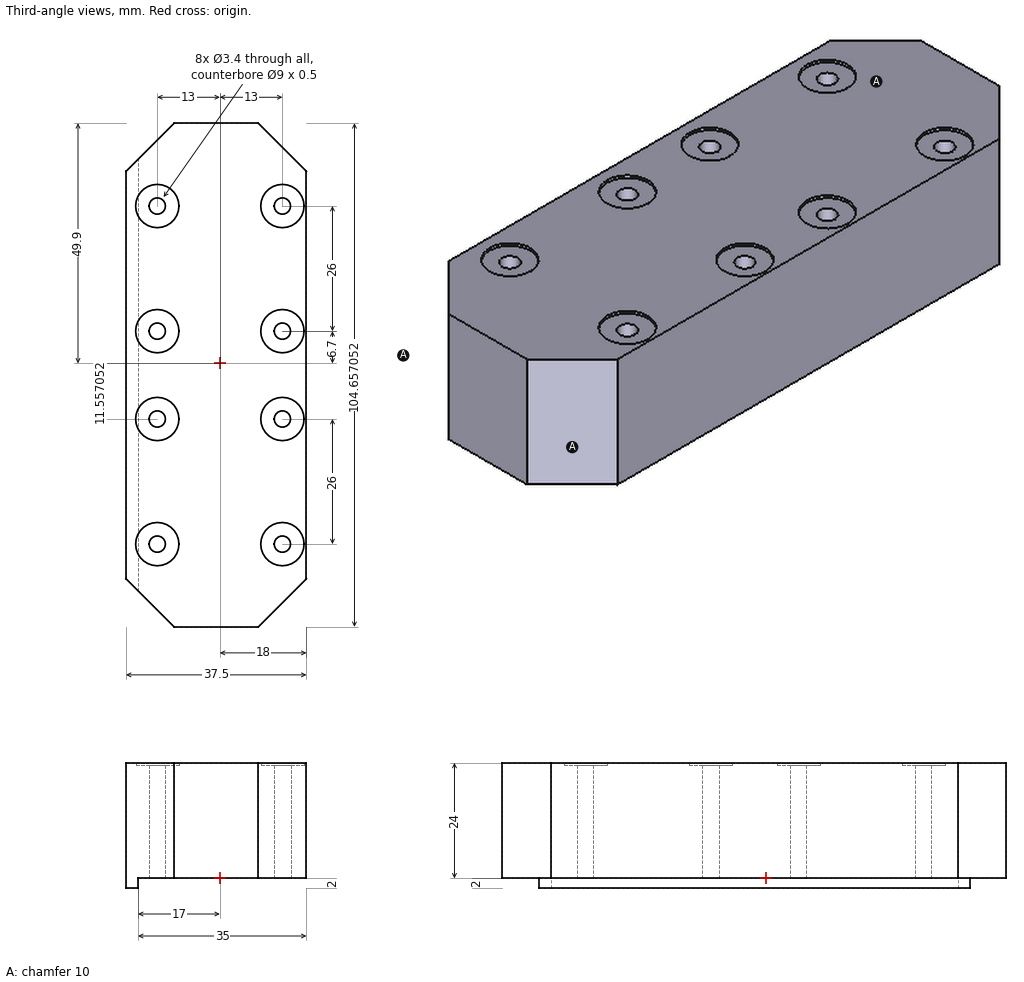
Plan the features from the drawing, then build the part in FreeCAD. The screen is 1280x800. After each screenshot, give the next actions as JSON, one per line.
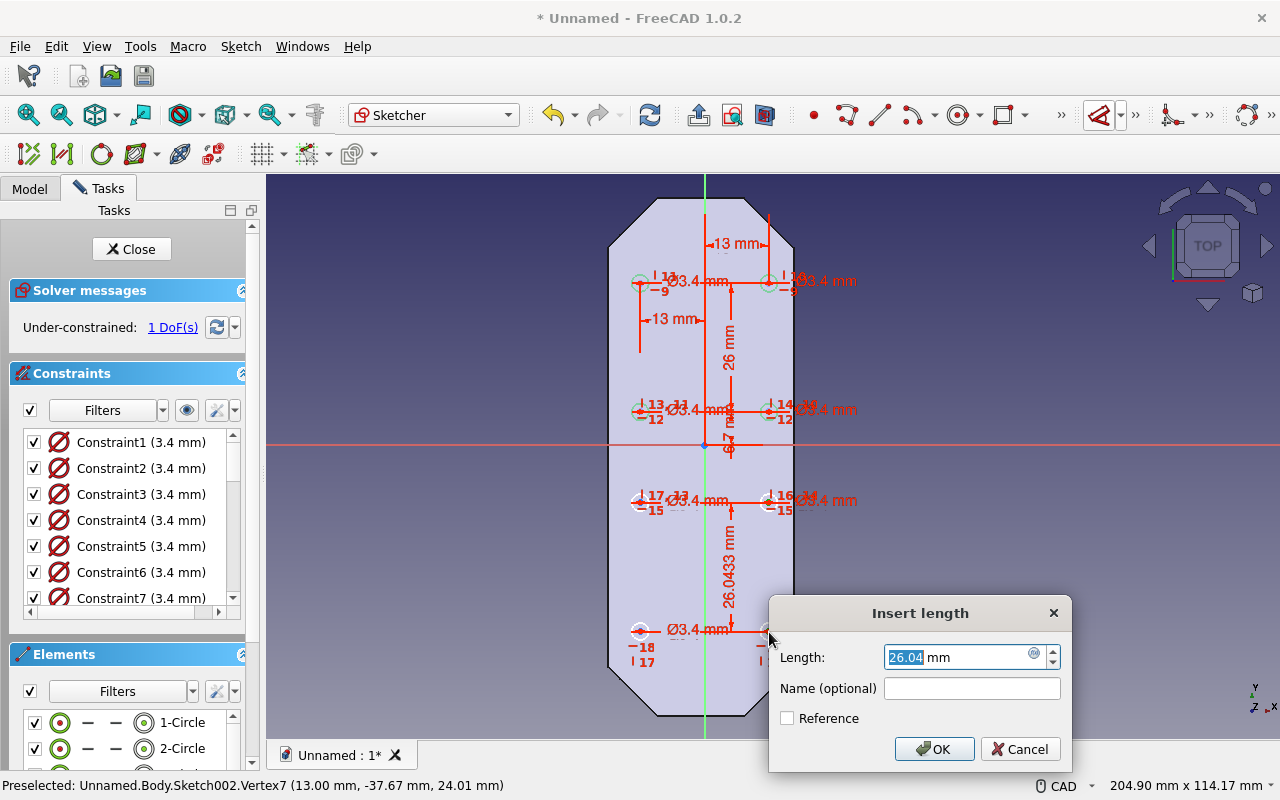
{"action": "type", "text": "26"}
{"action": "key", "text": "Return"}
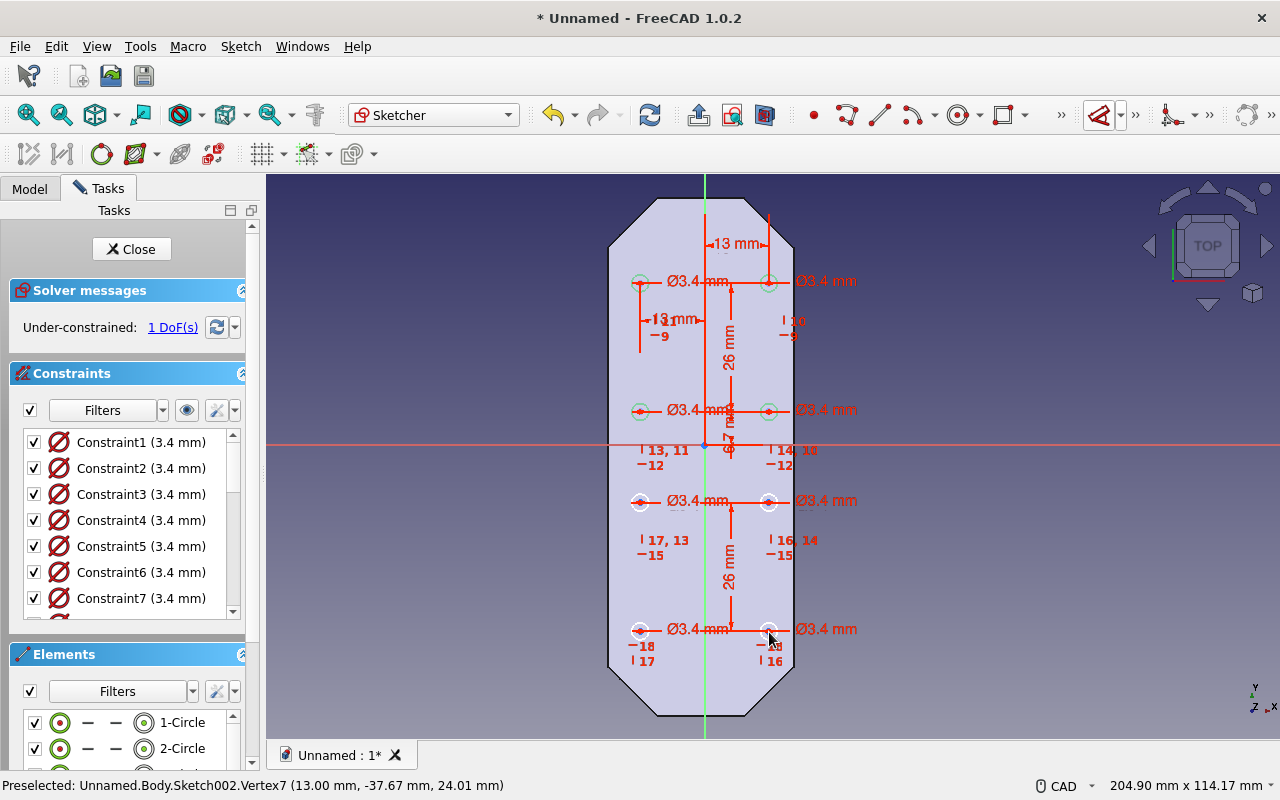
{"action": "left_click", "coordinate": [640, 503]}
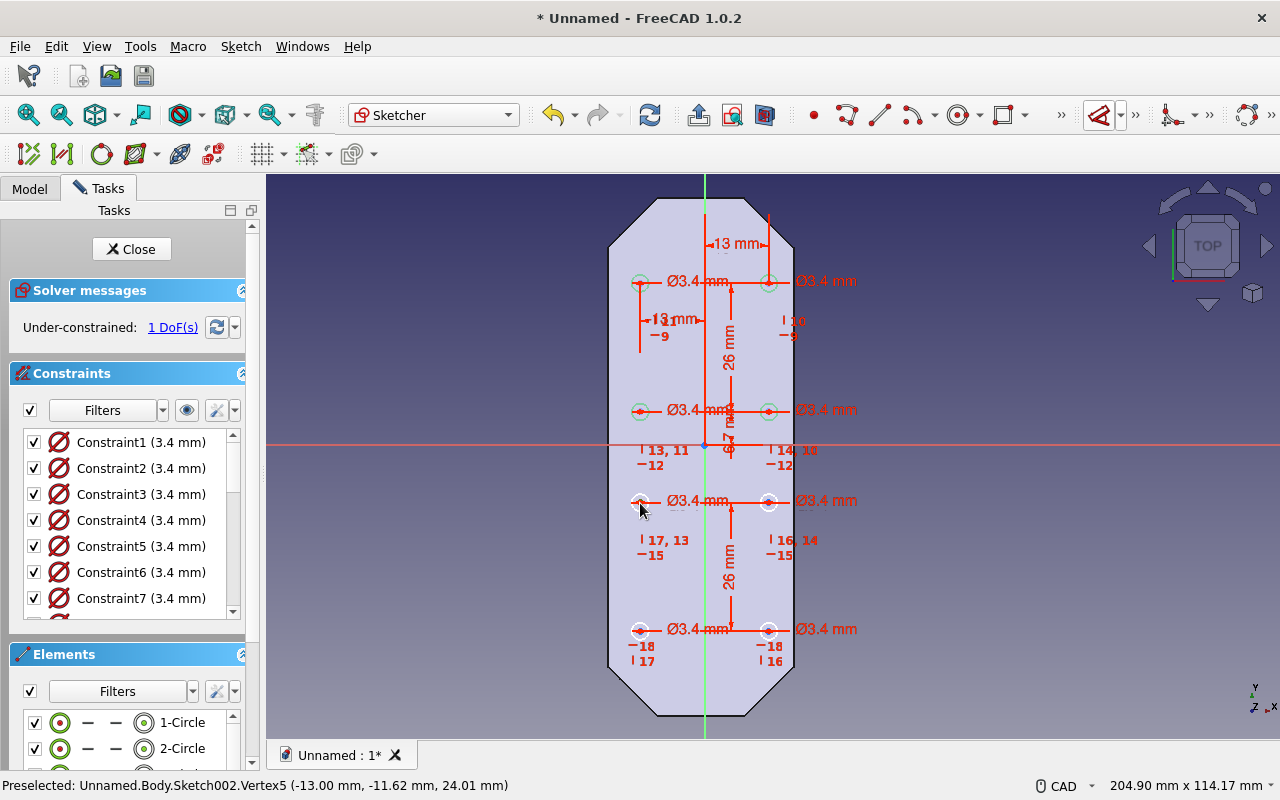
{"action": "left_click", "coordinate": [1120, 116]}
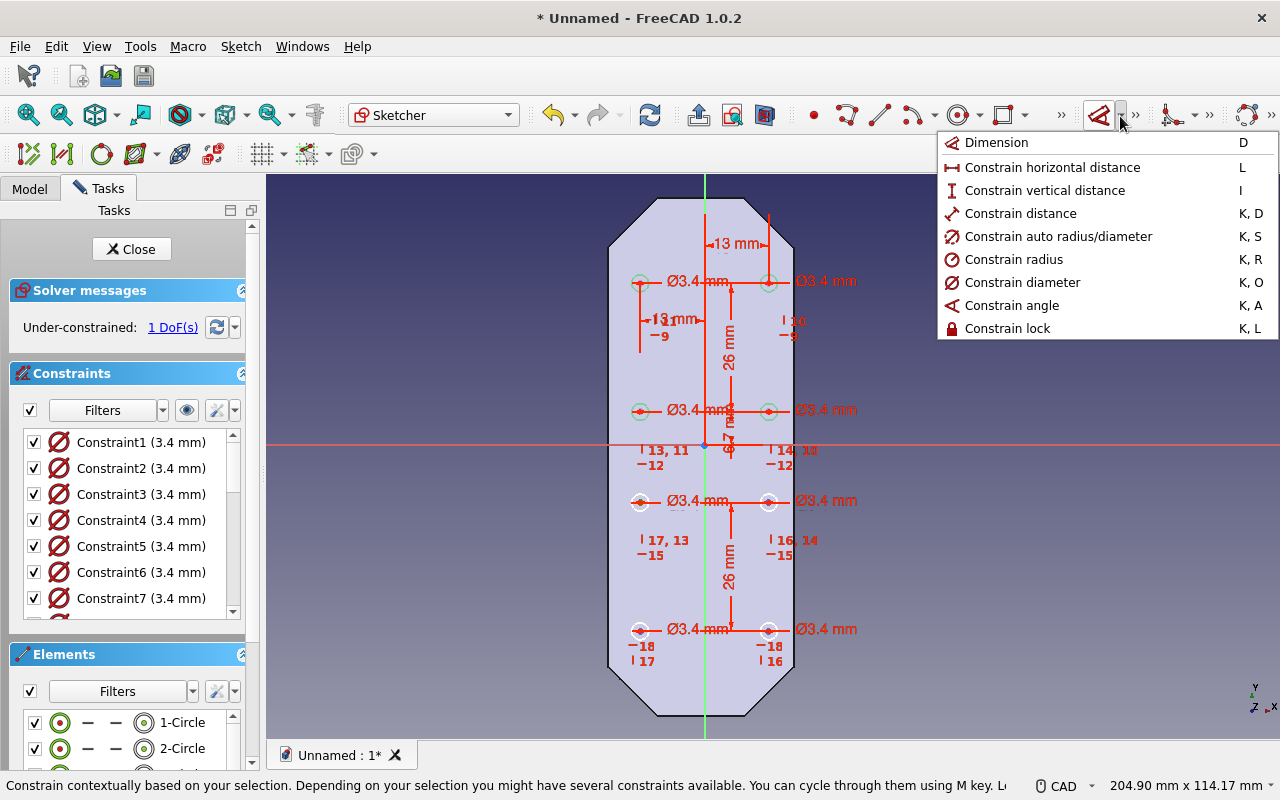
{"action": "left_click", "coordinate": [1108, 190]}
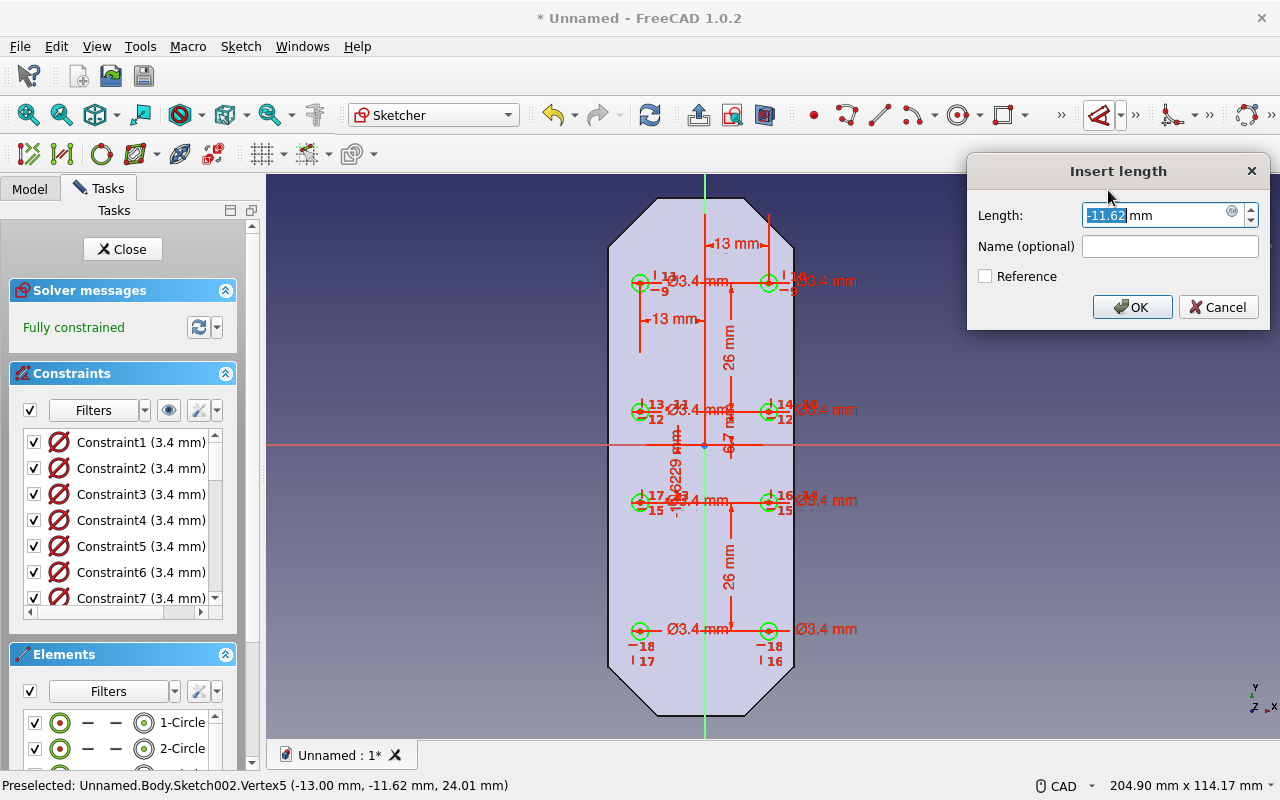
{"action": "type", "text": "-11.557052"}
{"action": "key", "text": "Return"}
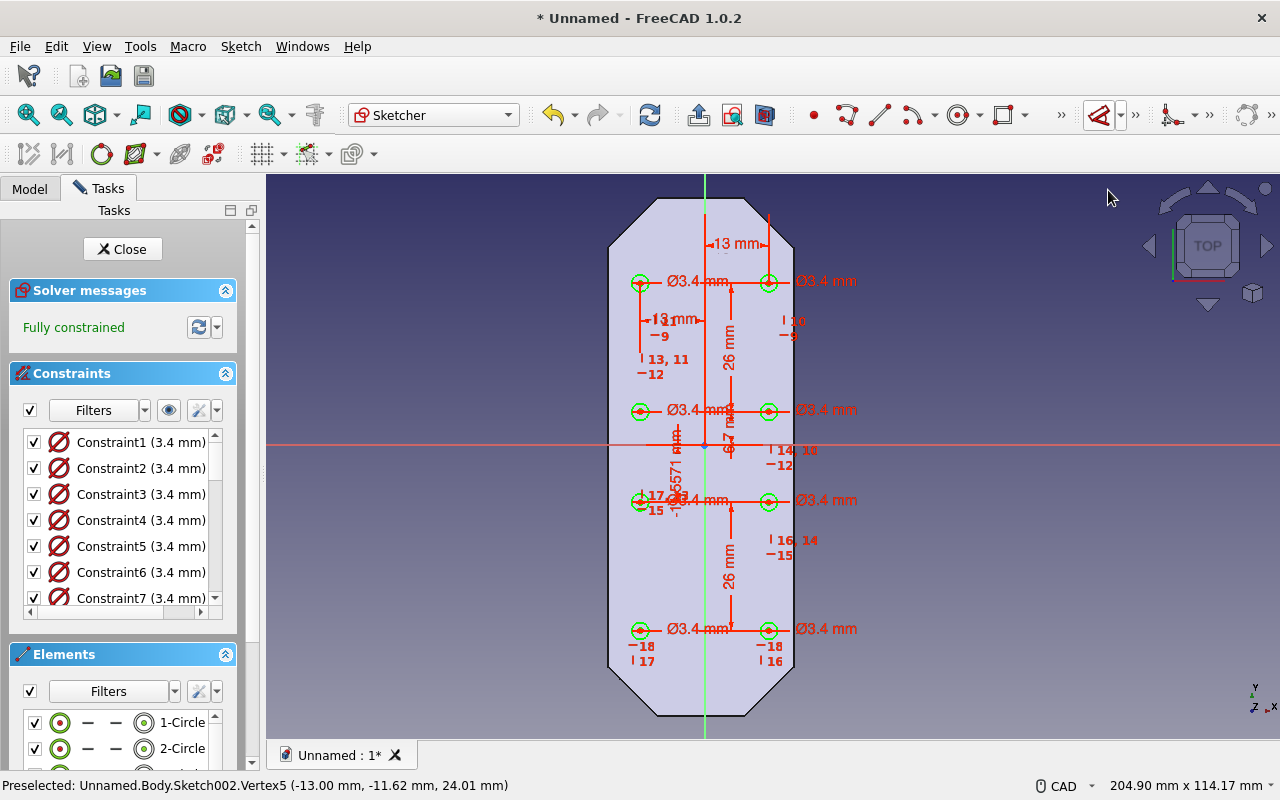
{"action": "left_click", "coordinate": [123, 249]}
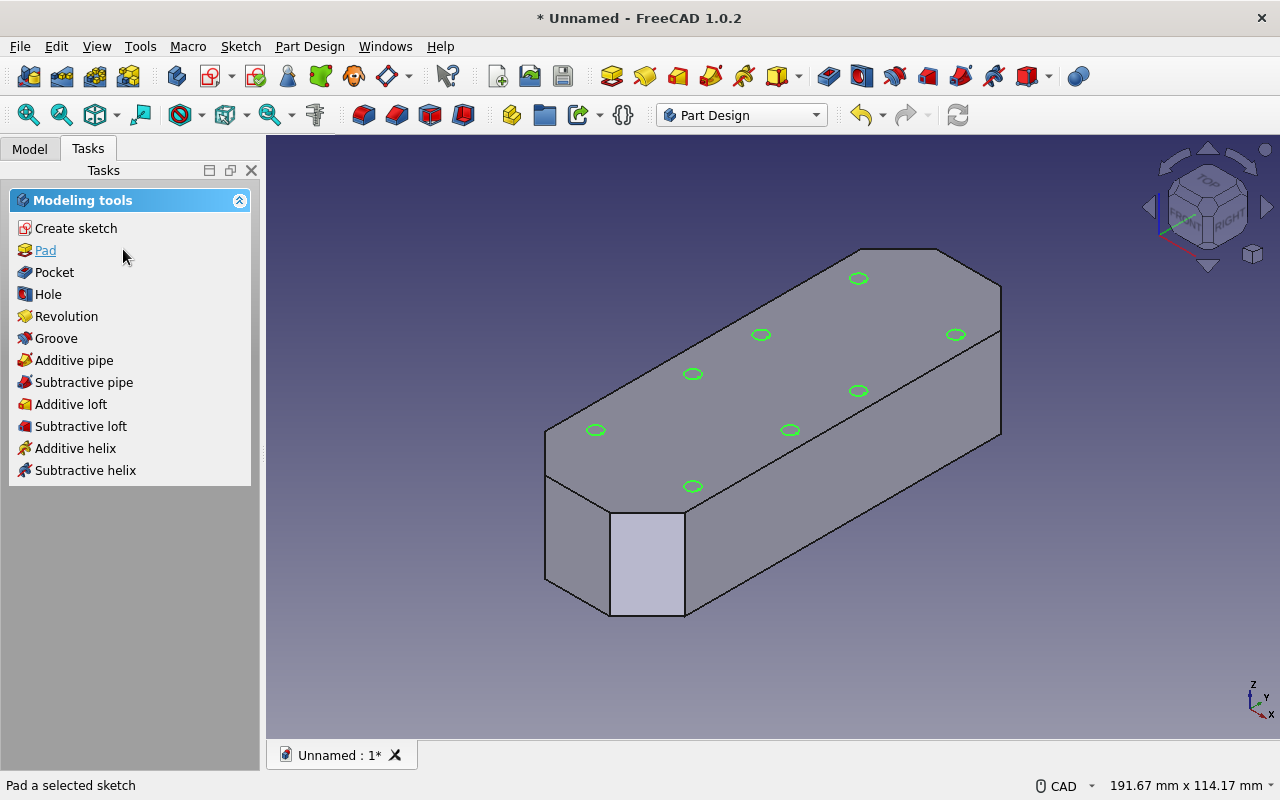
{"action": "left_click", "coordinate": [862, 76]}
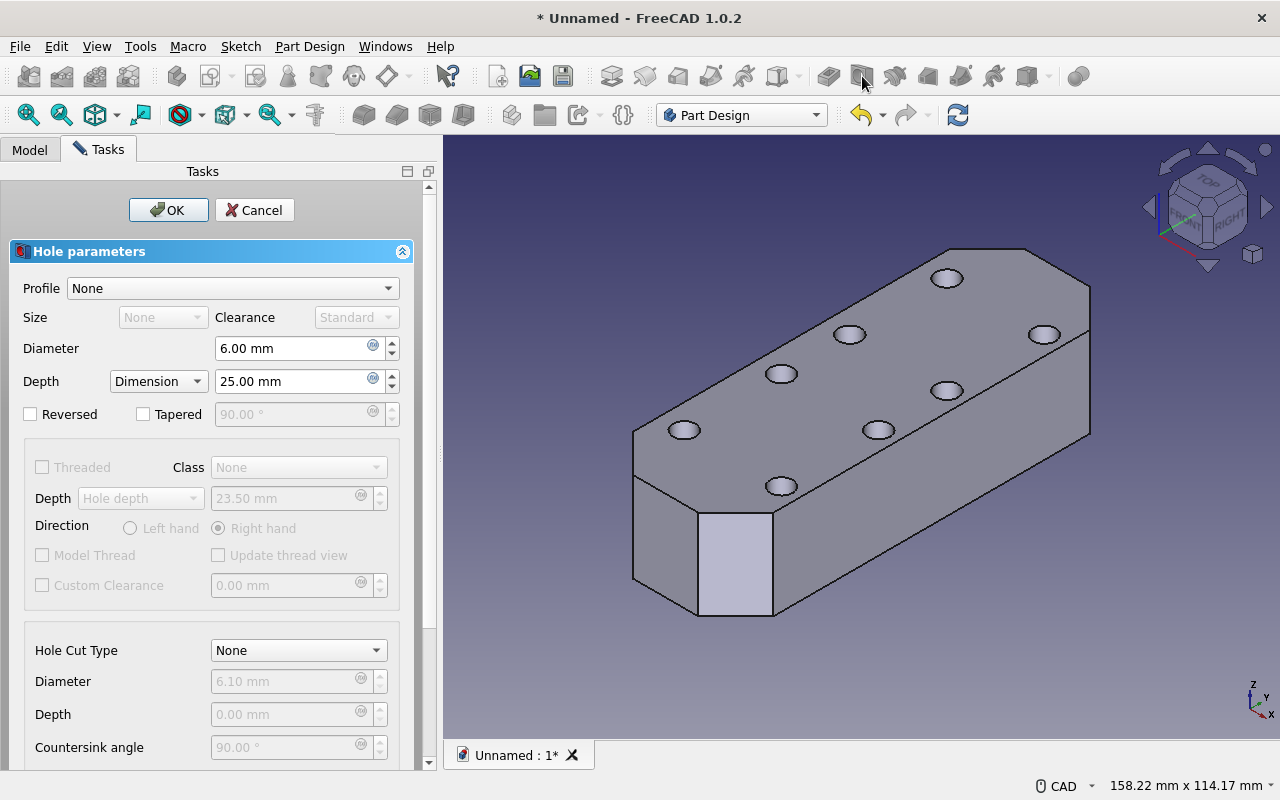
{"action": "triple_click", "coordinate": [300, 348]}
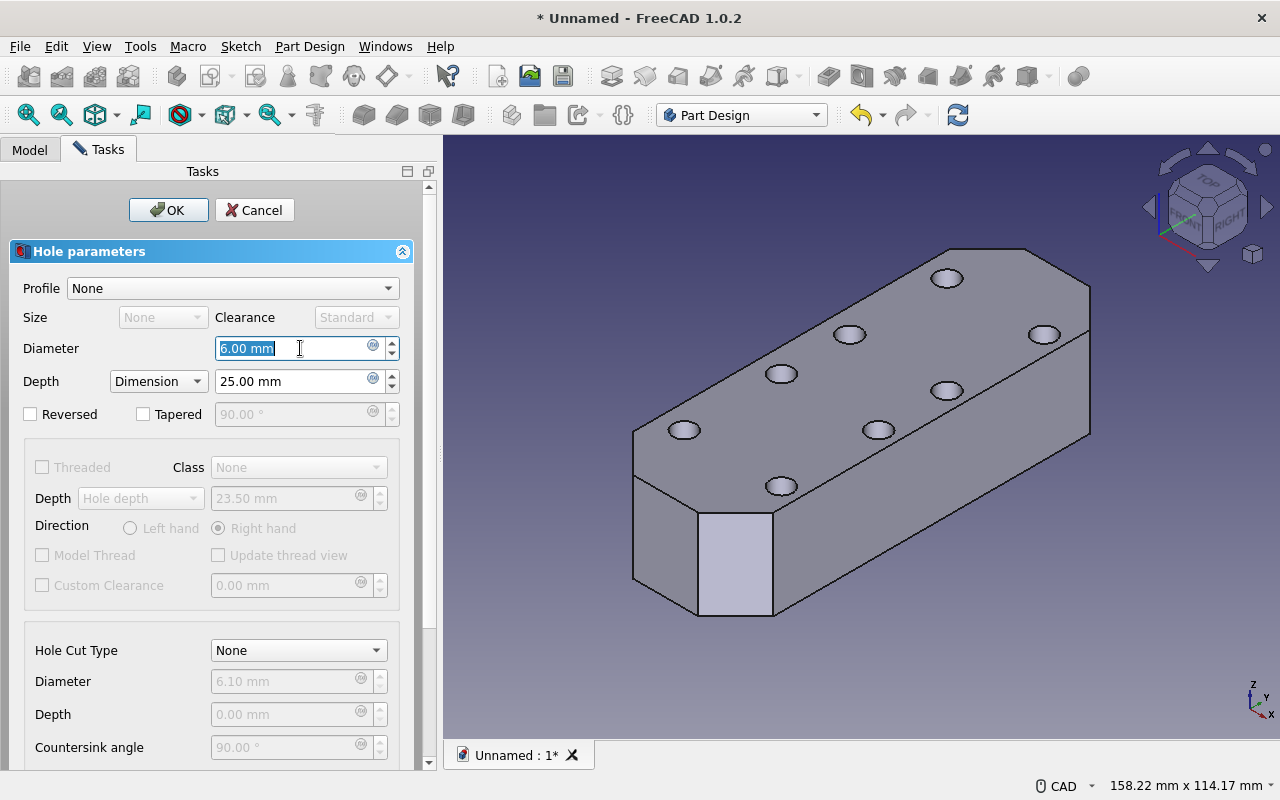
{"action": "type", "text": "3.4"}
{"action": "key", "text": "Tab"}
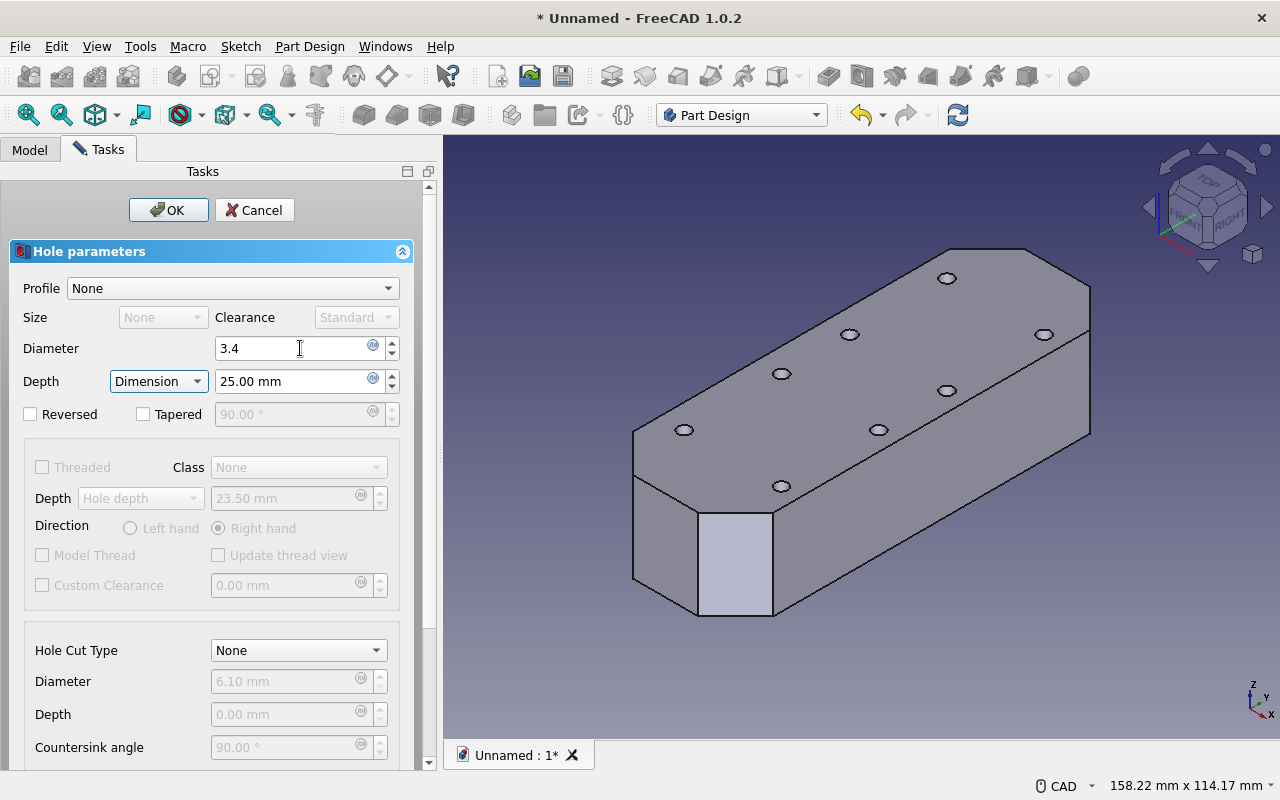
{"action": "left_click", "coordinate": [160, 382]}